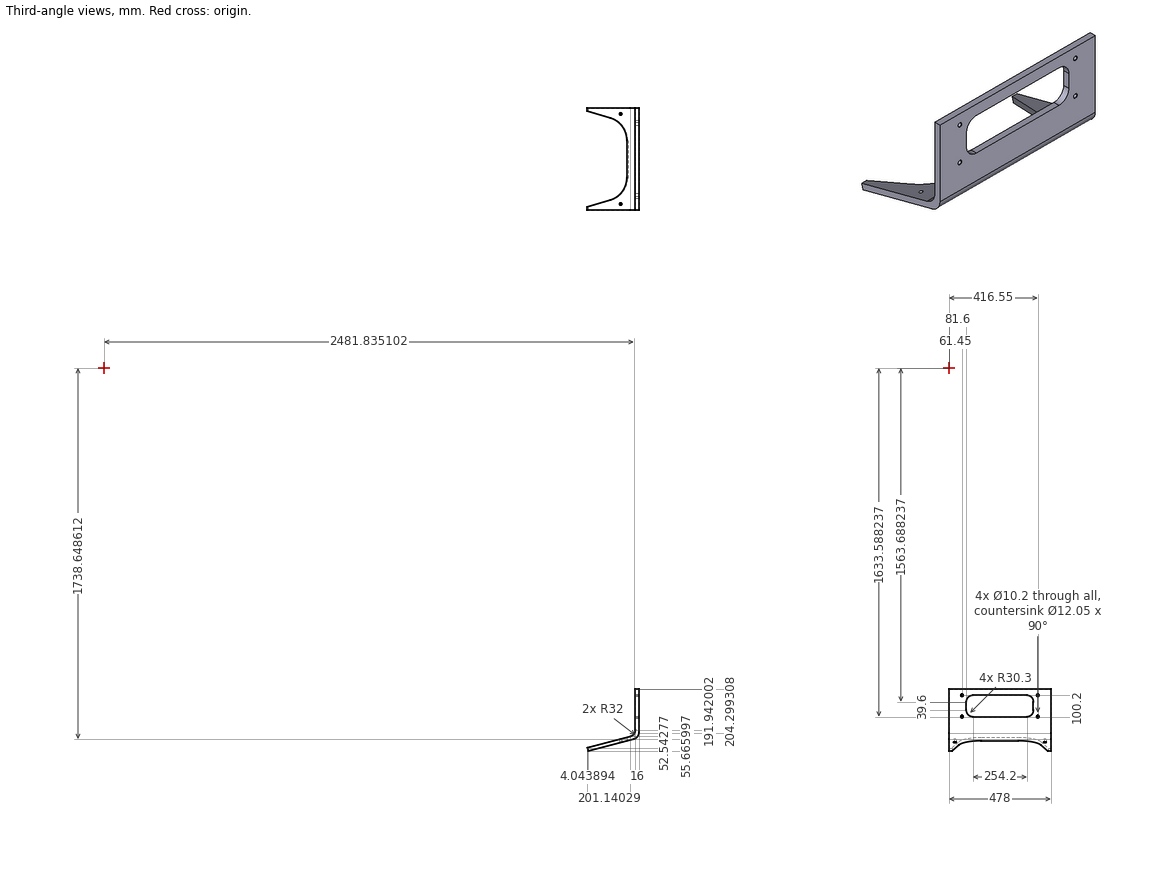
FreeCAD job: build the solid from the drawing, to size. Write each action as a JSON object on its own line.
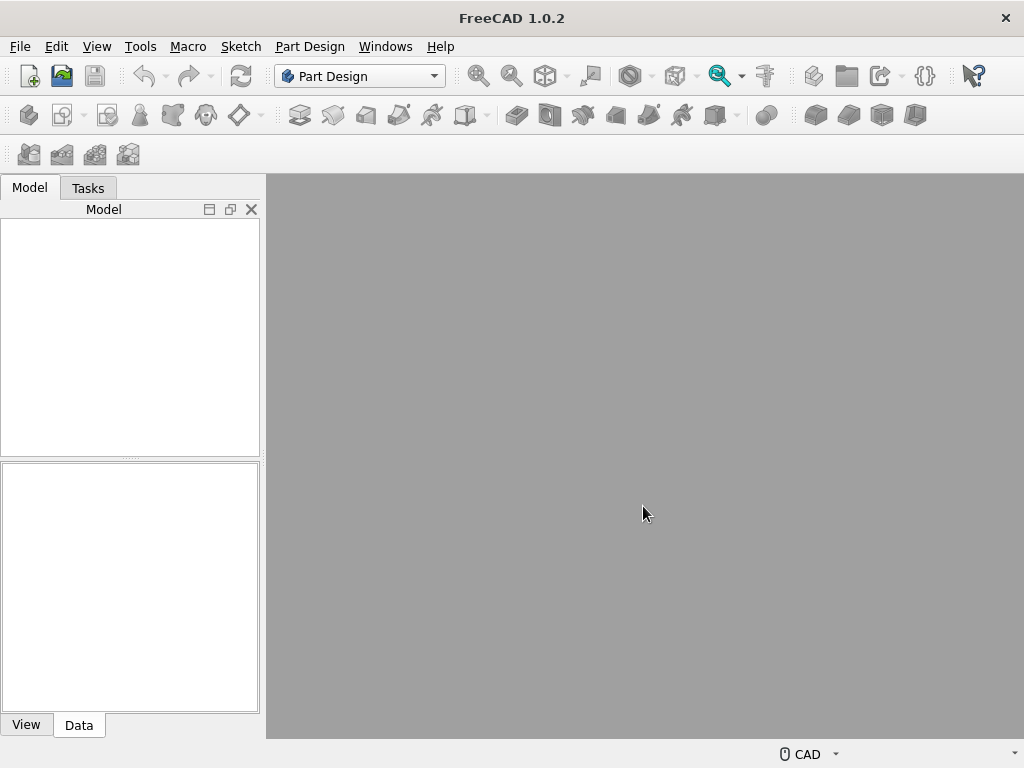
{"action": "left_click", "coordinate": [29, 76]}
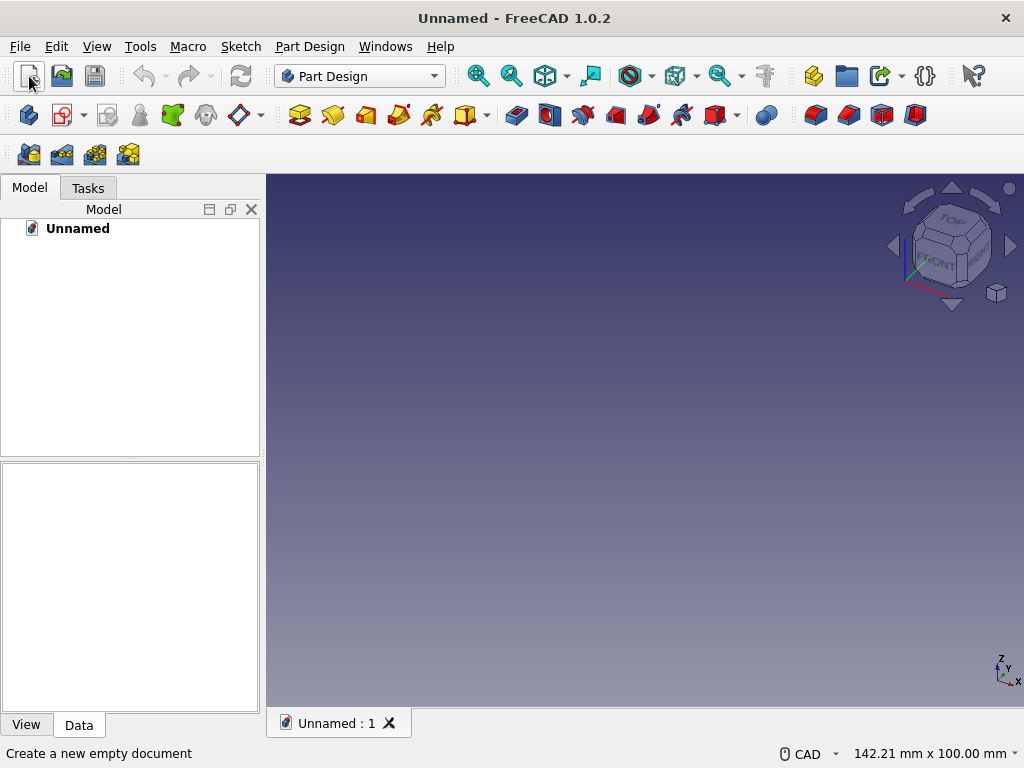
{"action": "left_click", "coordinate": [62, 116]}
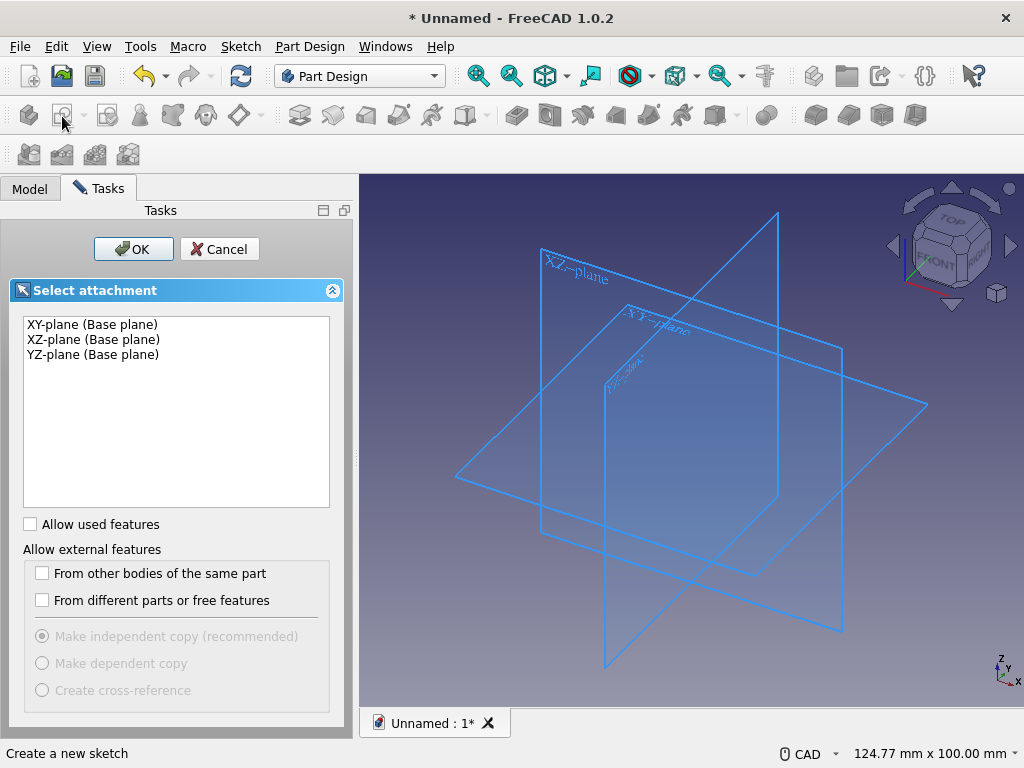
{"action": "left_click", "coordinate": [84, 340]}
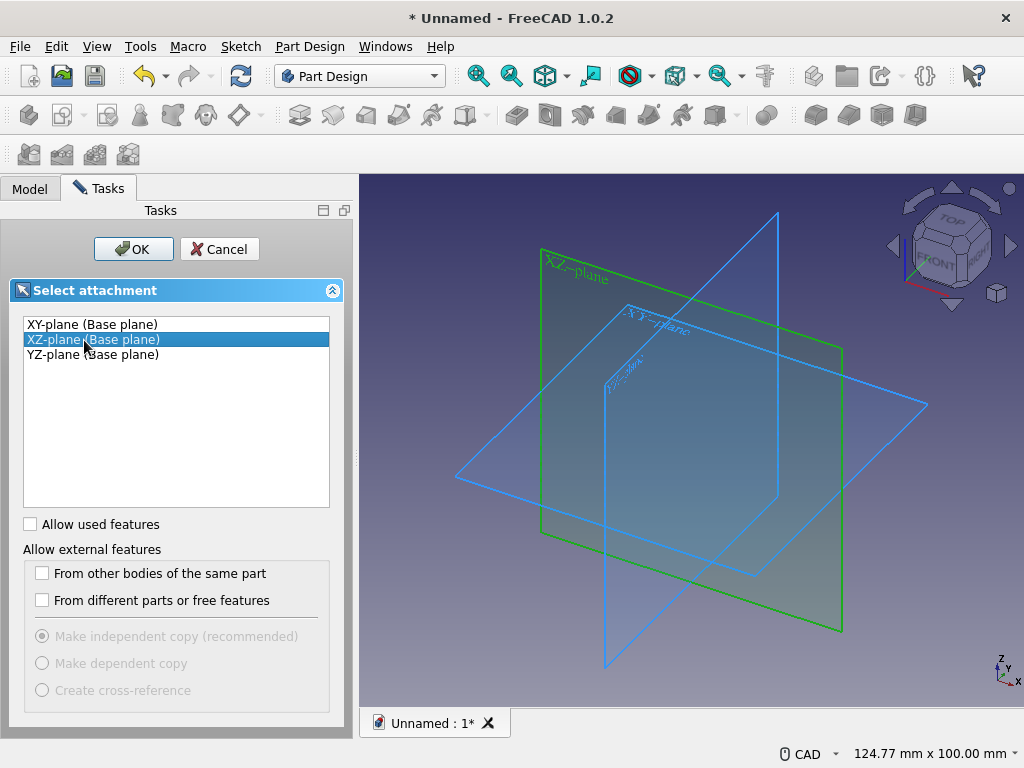
{"action": "left_click", "coordinate": [134, 249]}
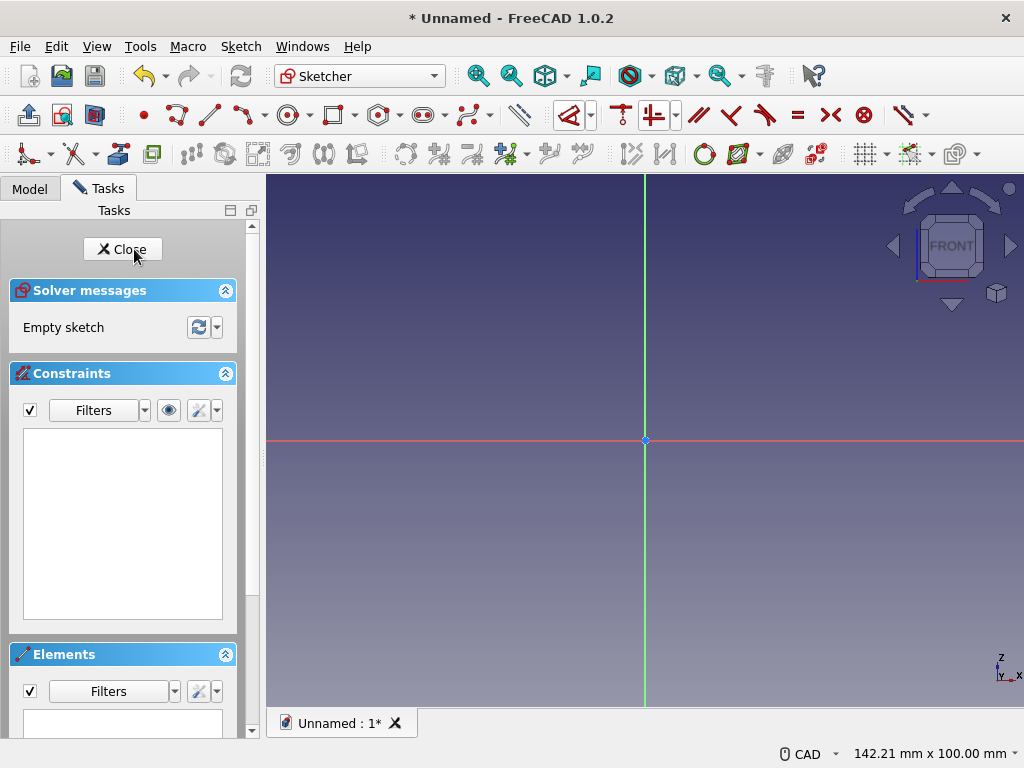
{"action": "scroll", "coordinate": [576, 440], "scroll_direction": "down", "scroll_amount": 8}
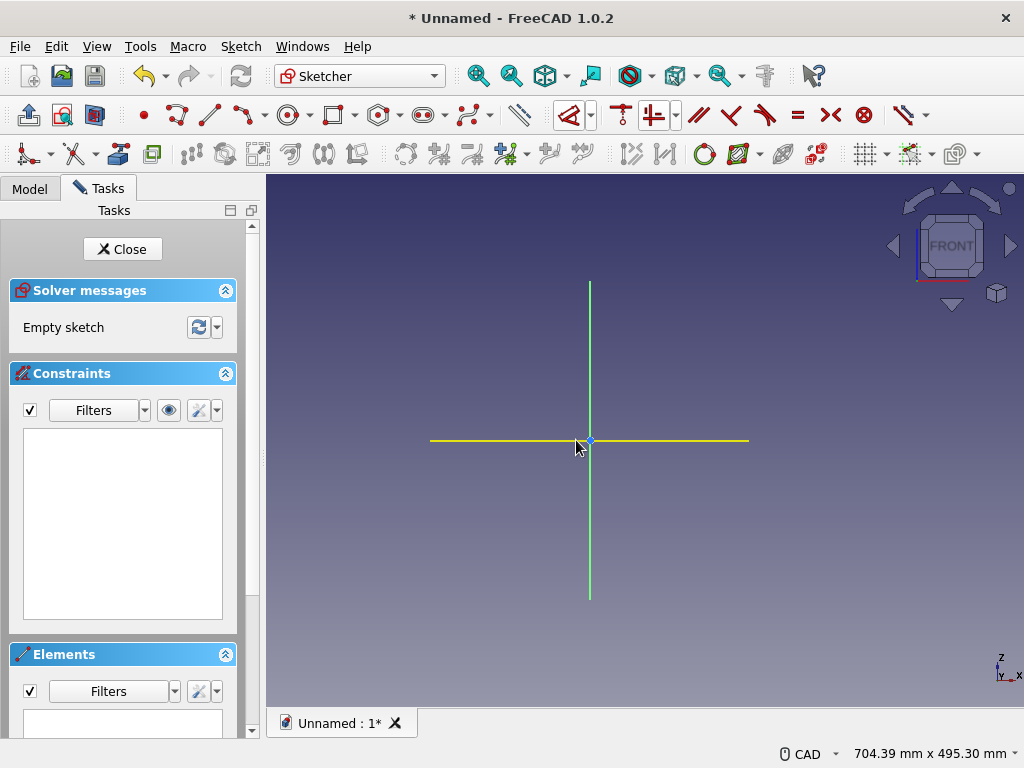
{"action": "scroll", "coordinate": [576, 440], "scroll_direction": "down", "scroll_amount": 5}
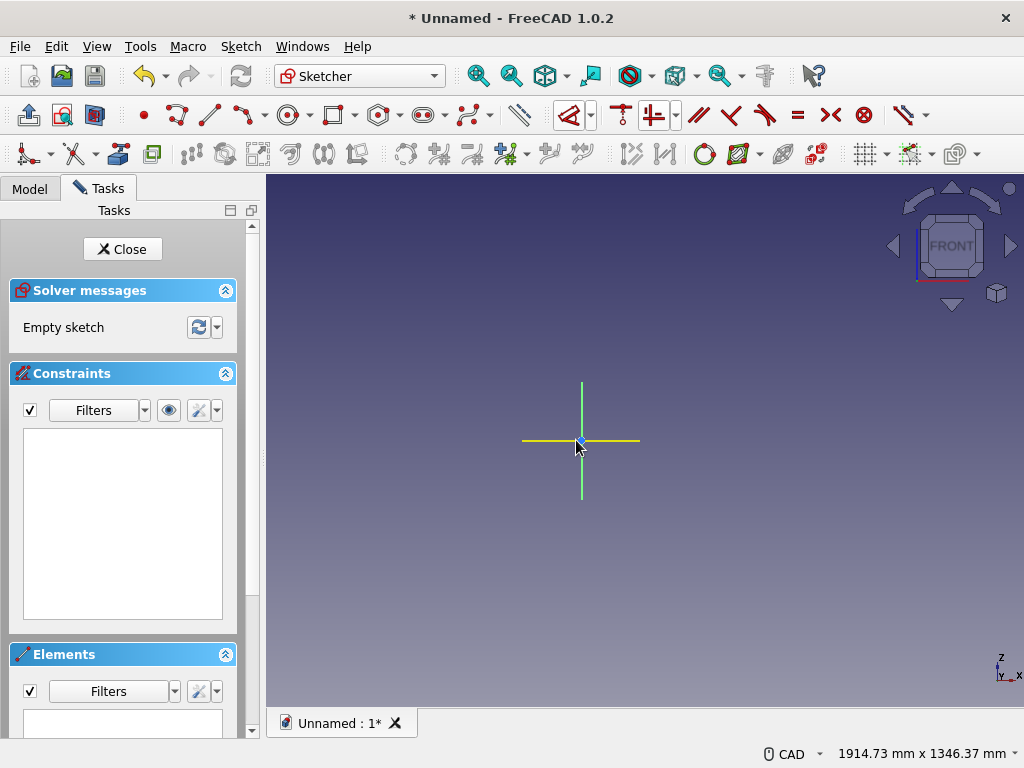
{"action": "scroll", "coordinate": [576, 440], "scroll_direction": "down", "scroll_amount": 5}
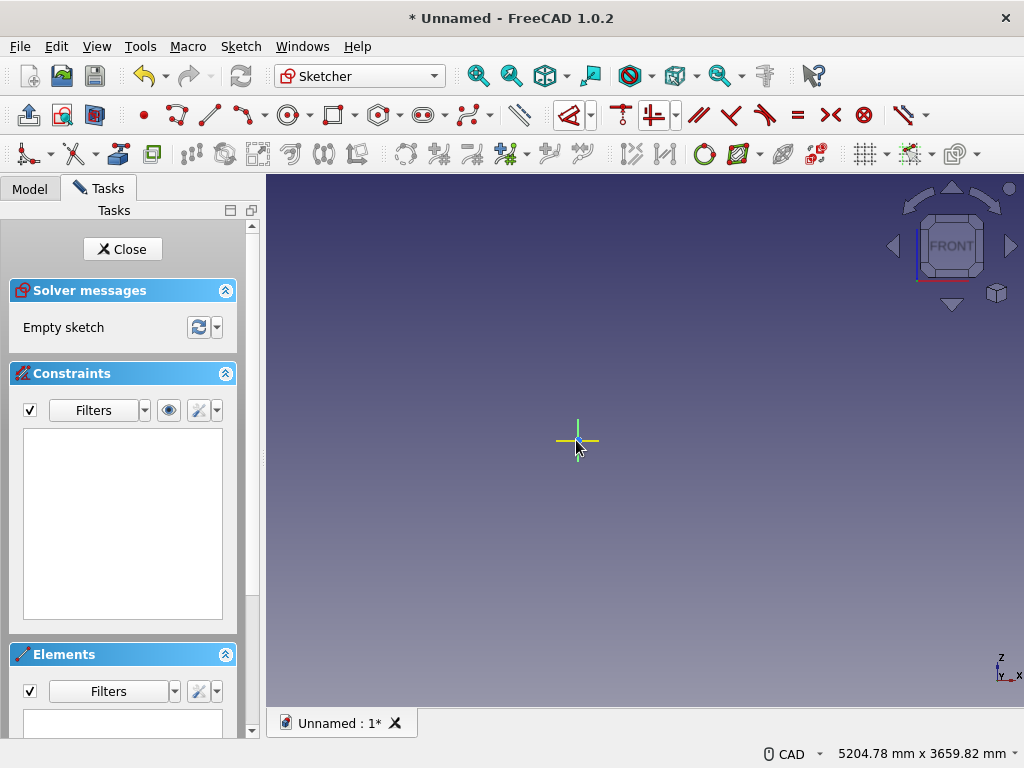
{"action": "scroll", "coordinate": [576, 440], "scroll_direction": "down", "scroll_amount": 5}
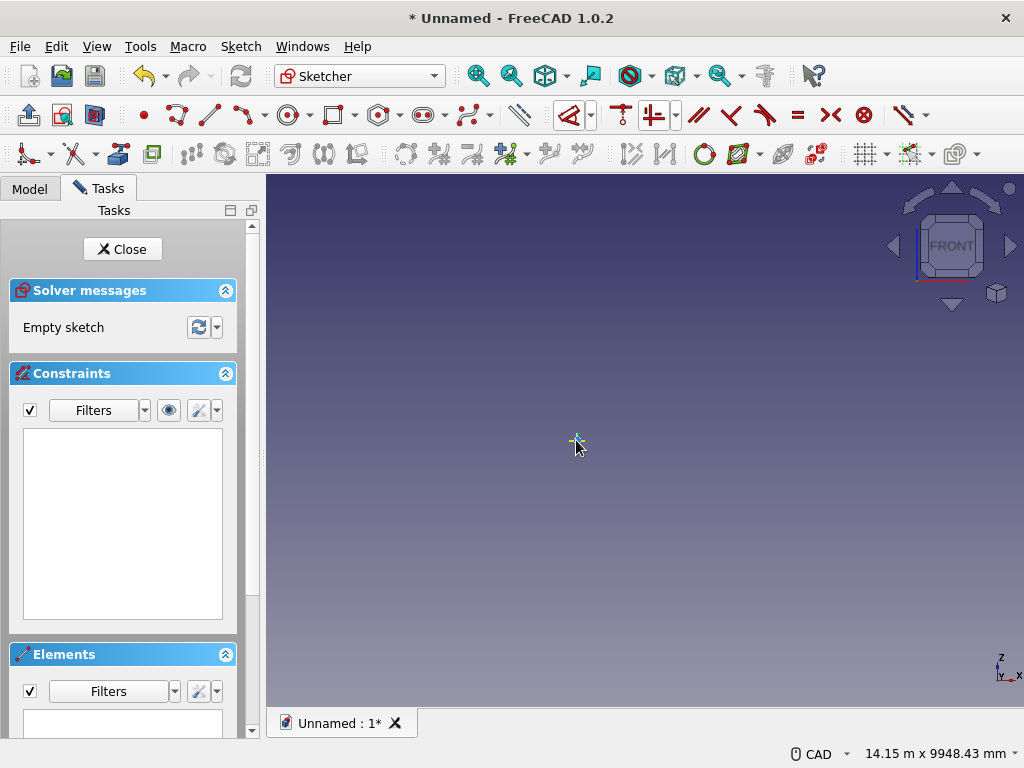
{"action": "scroll", "coordinate": [712, 533], "scroll_direction": "up", "scroll_amount": 15}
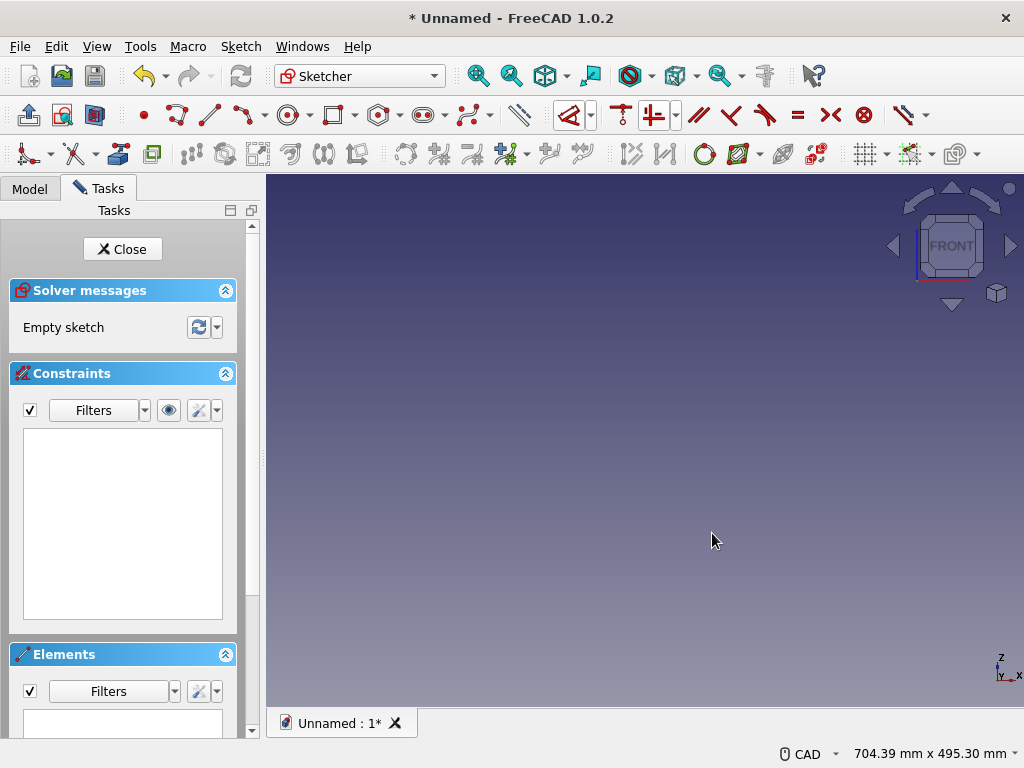
{"action": "left_click", "coordinate": [177, 116]}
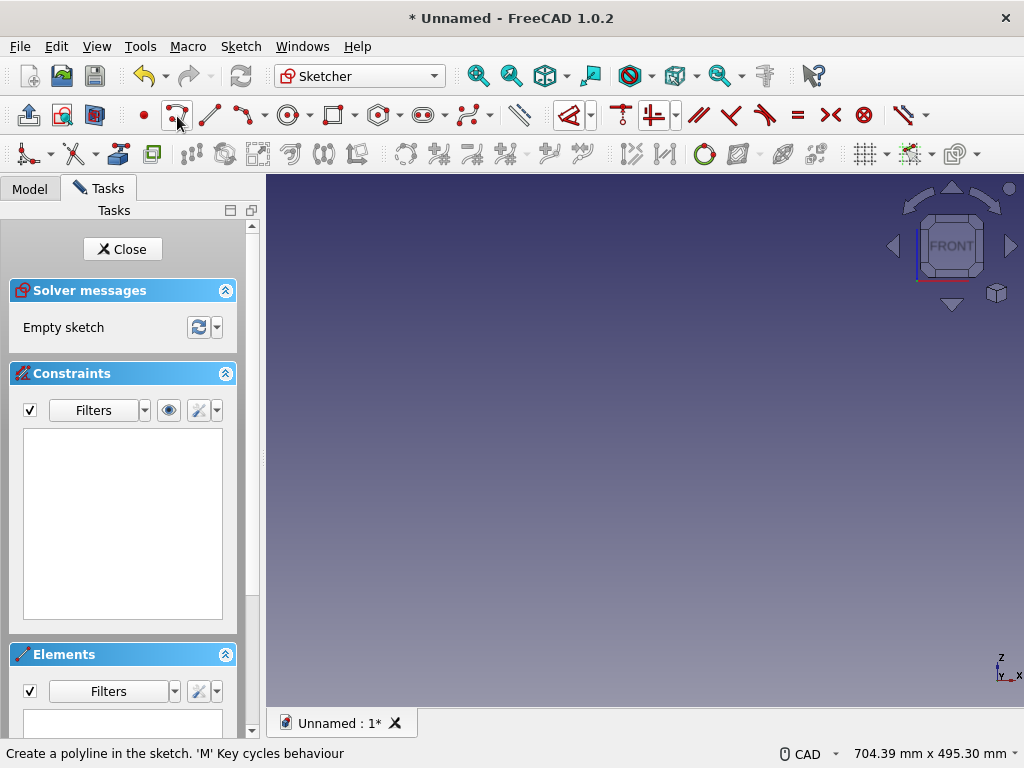
{"action": "left_click", "coordinate": [662, 533]}
{"action": "left_click", "coordinate": [433, 593]}
{"action": "left_click", "coordinate": [428, 576]}
{"action": "left_click", "coordinate": [645, 520]}
{"action": "right_click", "coordinate": [645, 520]}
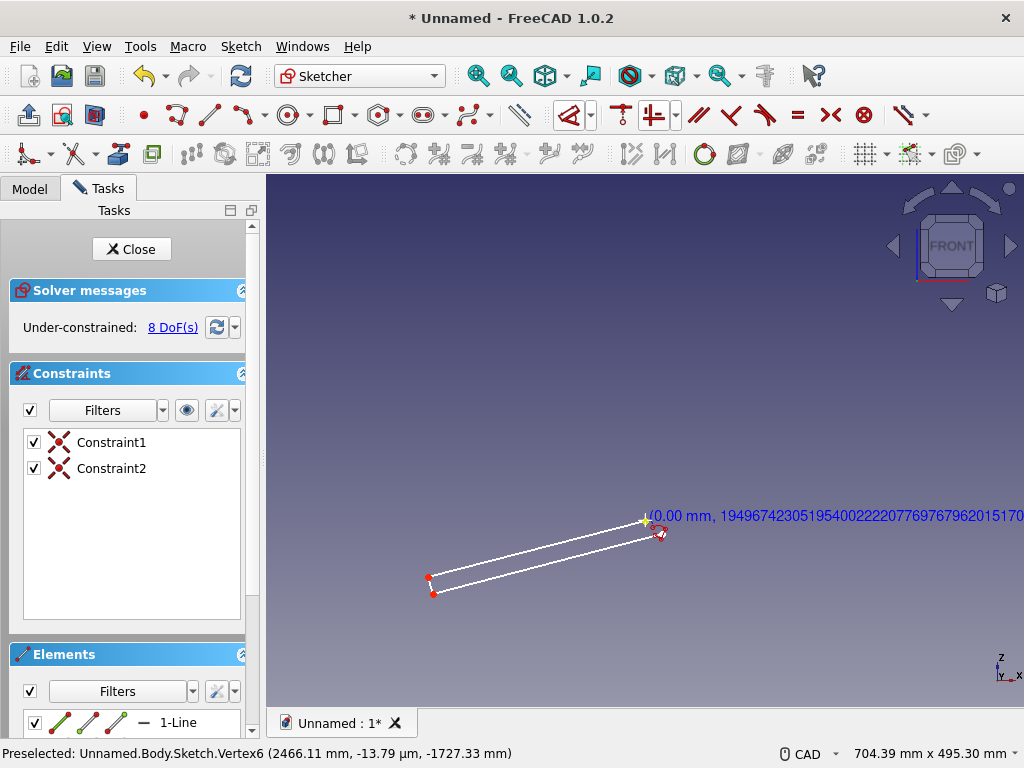
{"action": "left_click", "coordinate": [670, 487]}
{"action": "left_click", "coordinate": [670, 280]}
{"action": "left_click", "coordinate": [688, 280]}
{"action": "left_click", "coordinate": [688, 500]}
{"action": "right_click", "coordinate": [688, 500]}